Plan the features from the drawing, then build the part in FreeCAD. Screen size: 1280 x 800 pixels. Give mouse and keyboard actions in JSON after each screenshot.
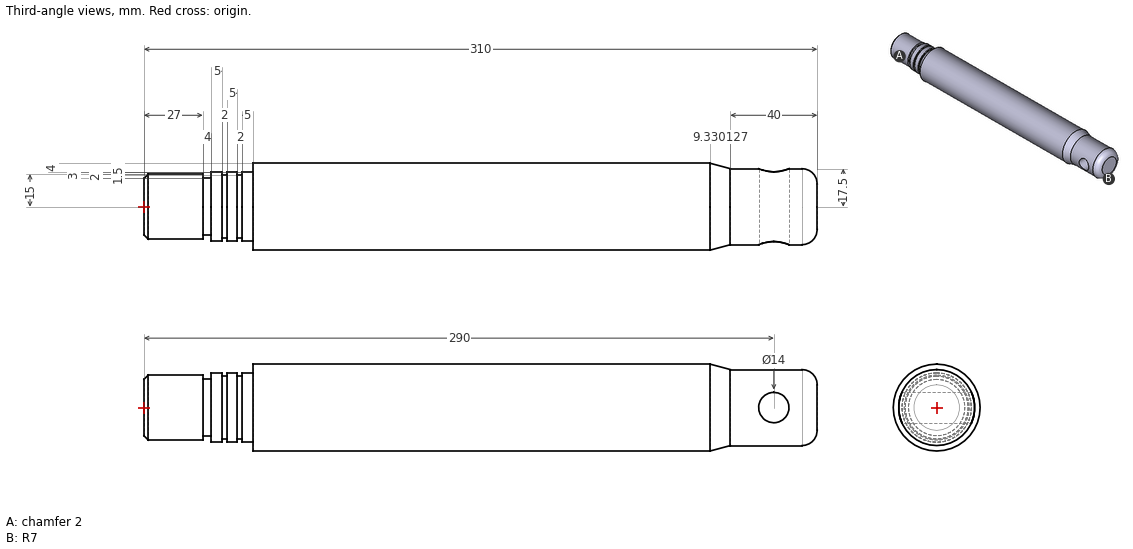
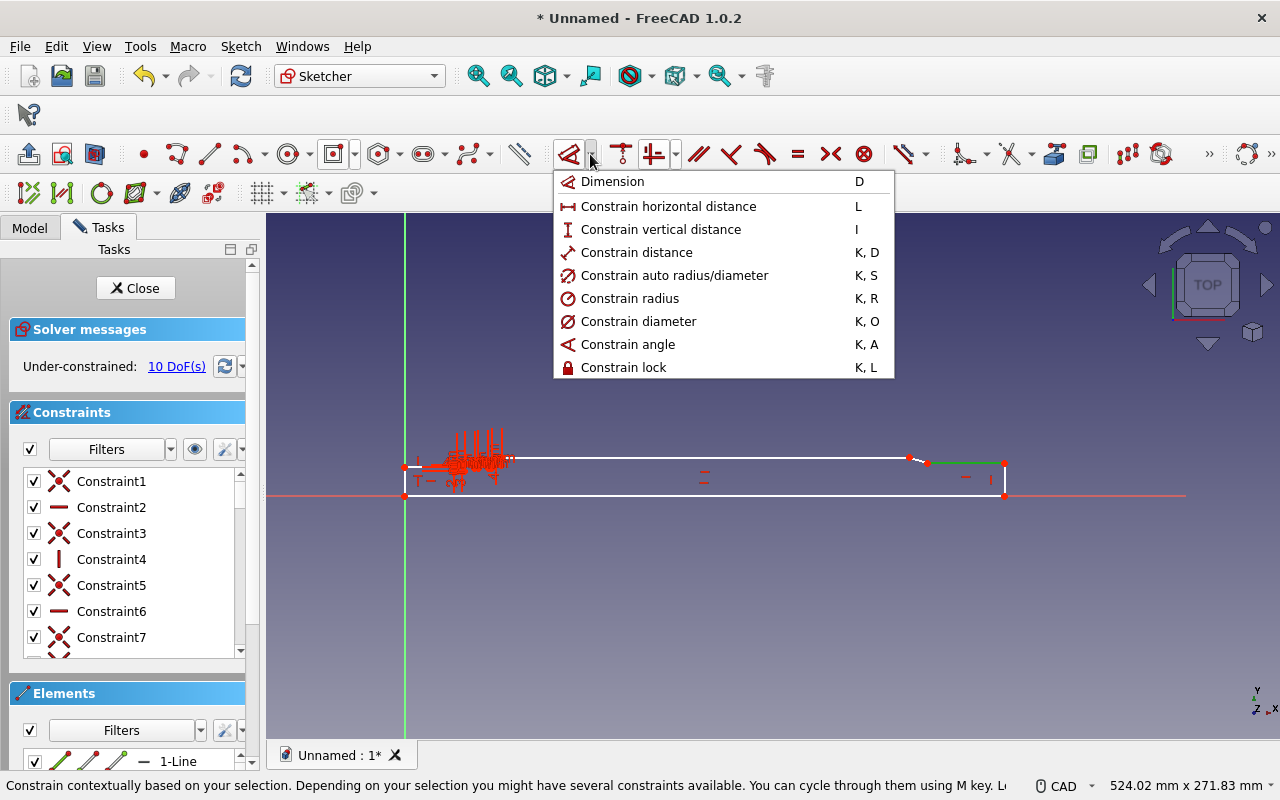
{"action": "left_click", "coordinate": [724, 206]}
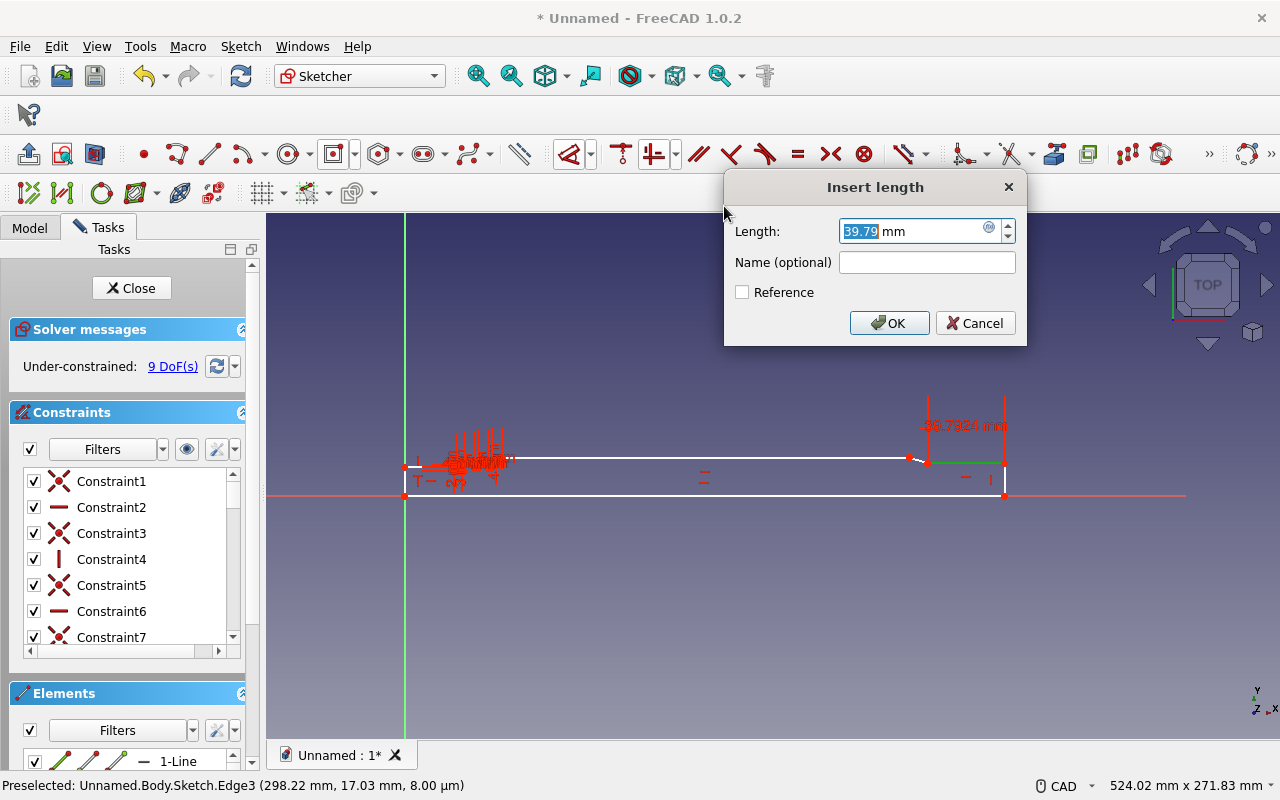
{"action": "type", "text": "40"}
{"action": "key", "text": "Return"}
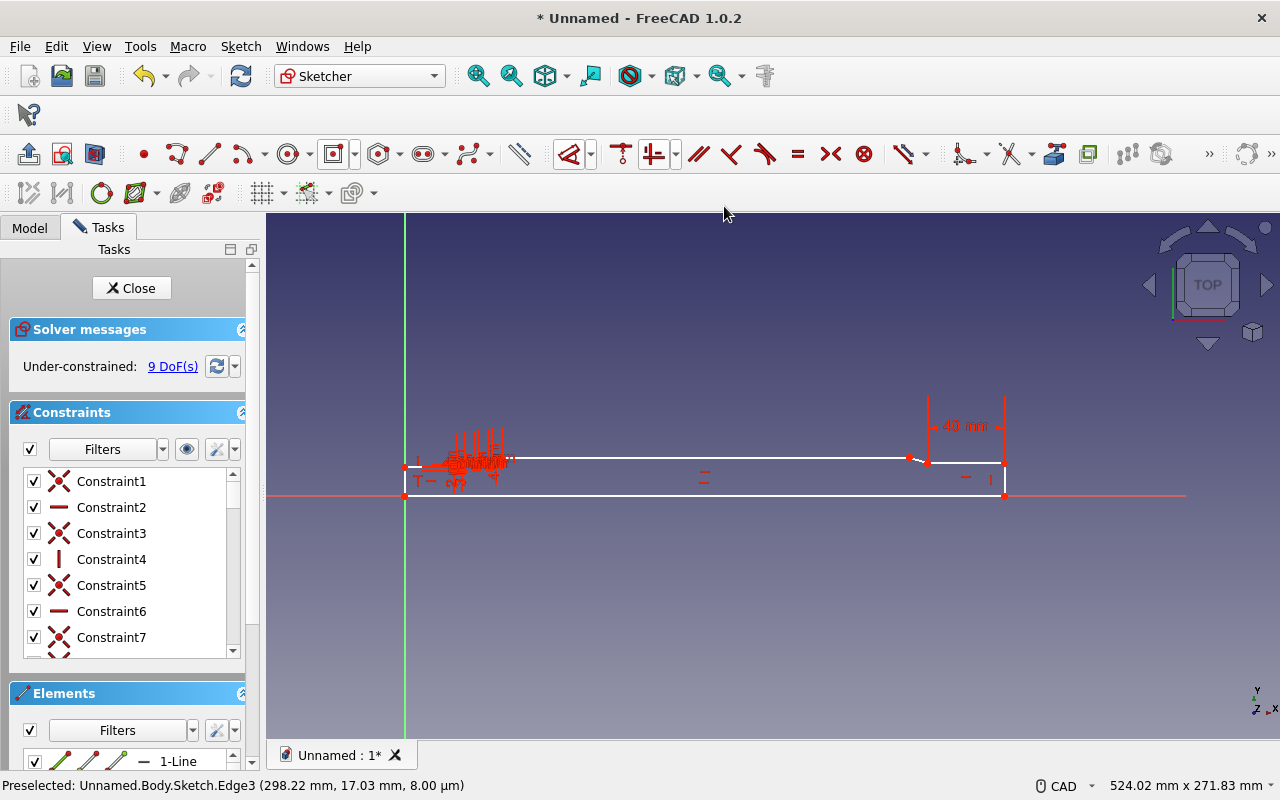
{"action": "scroll", "coordinate": [441, 467], "scroll_direction": "up", "scroll_amount": 4}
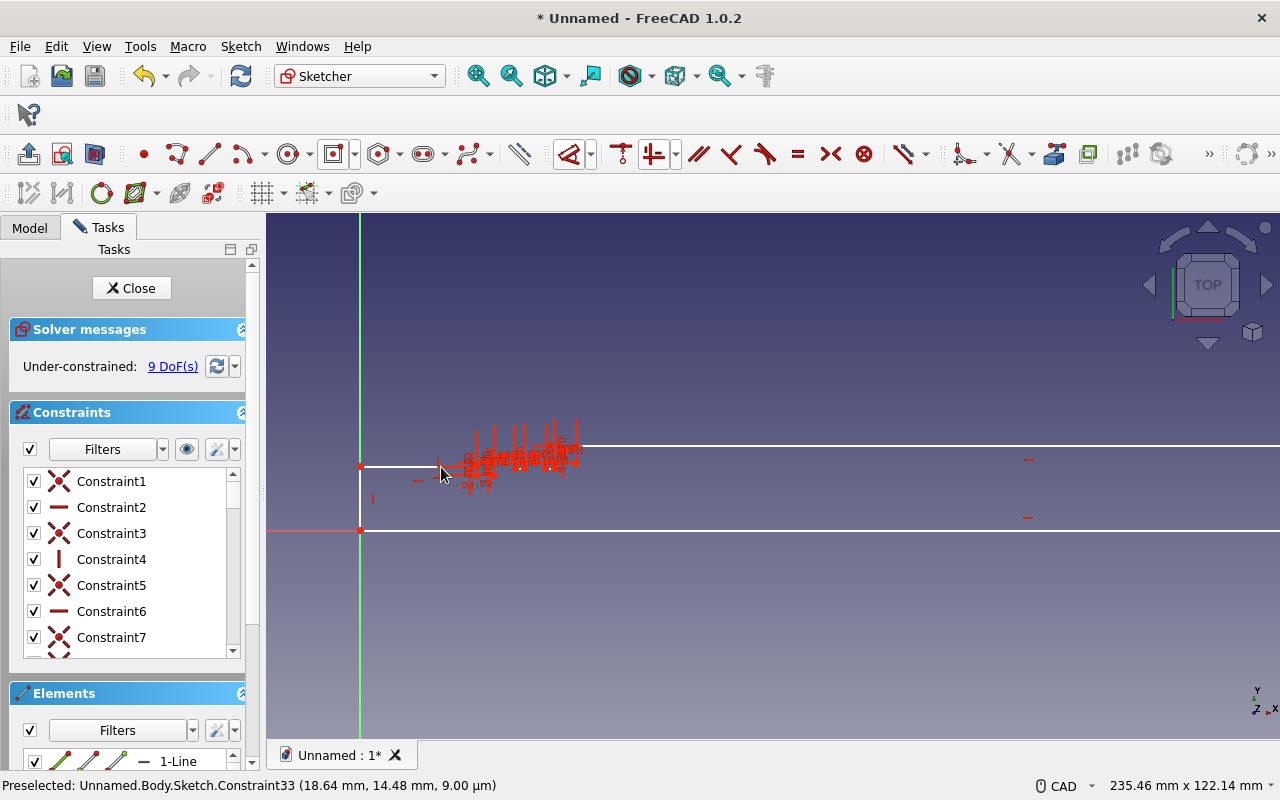
{"action": "left_click", "coordinate": [395, 467]}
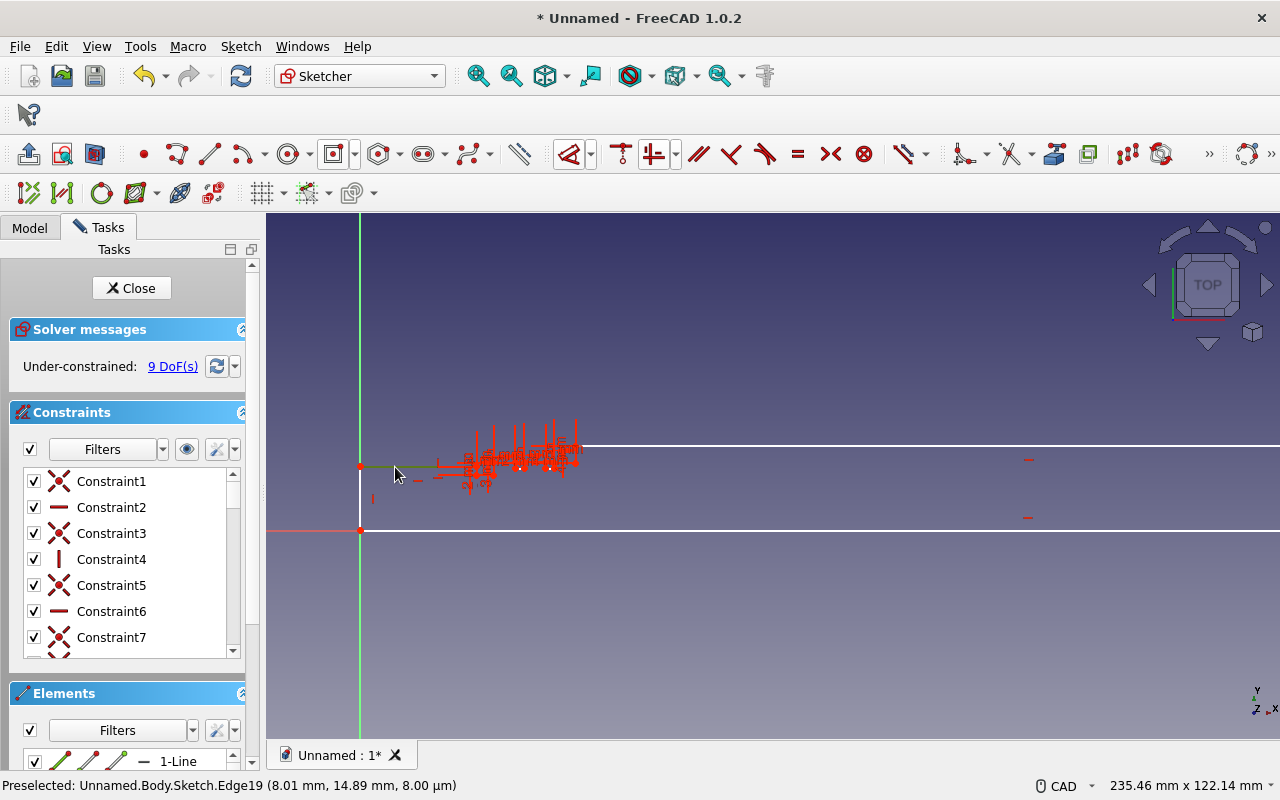
{"action": "left_click", "coordinate": [590, 154]}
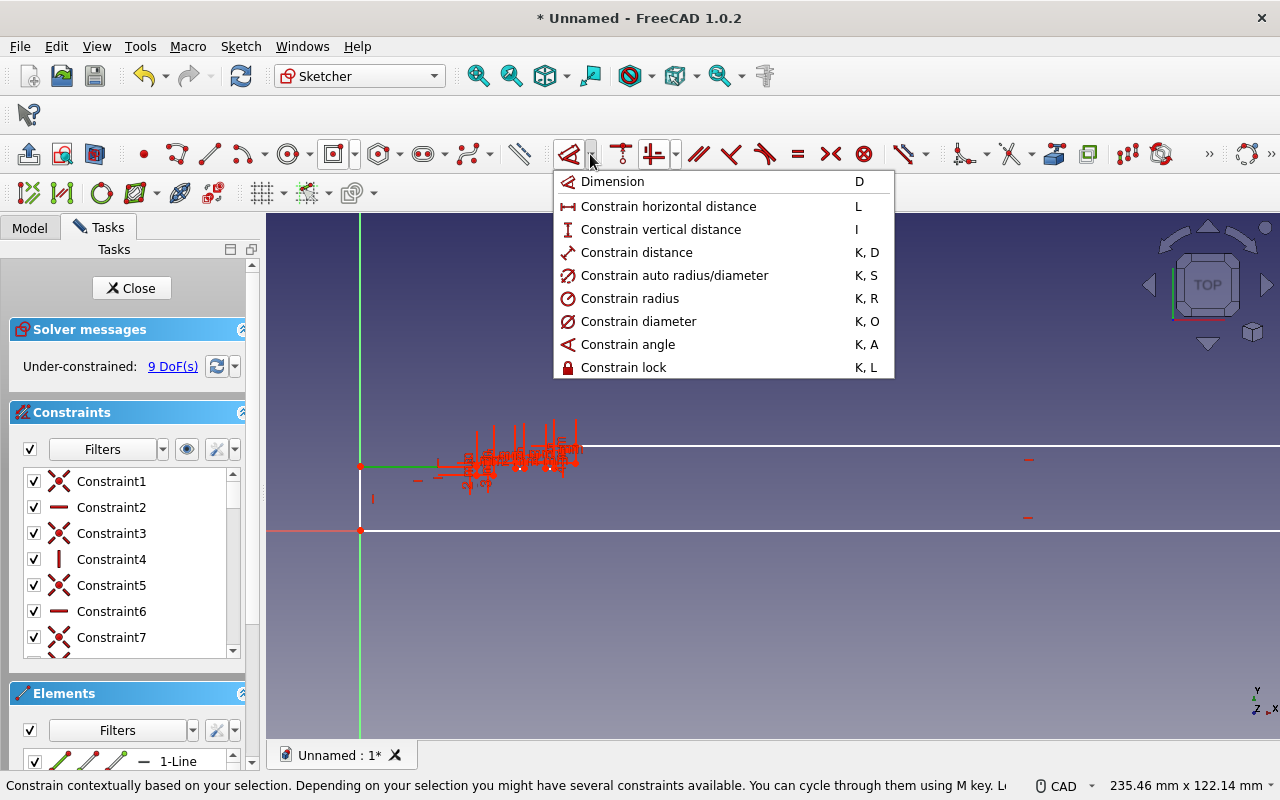
{"action": "left_click", "coordinate": [724, 206]}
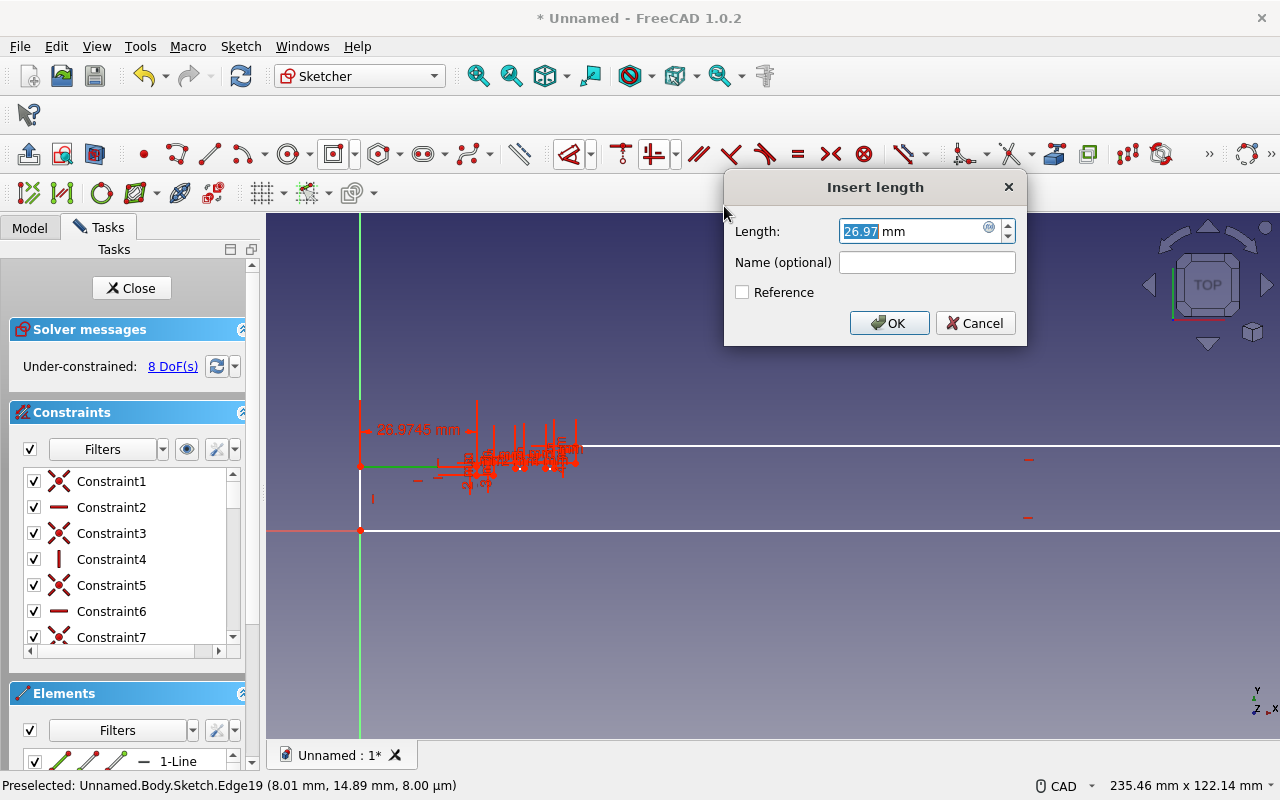
{"action": "type", "text": "27"}
{"action": "key", "text": "Return"}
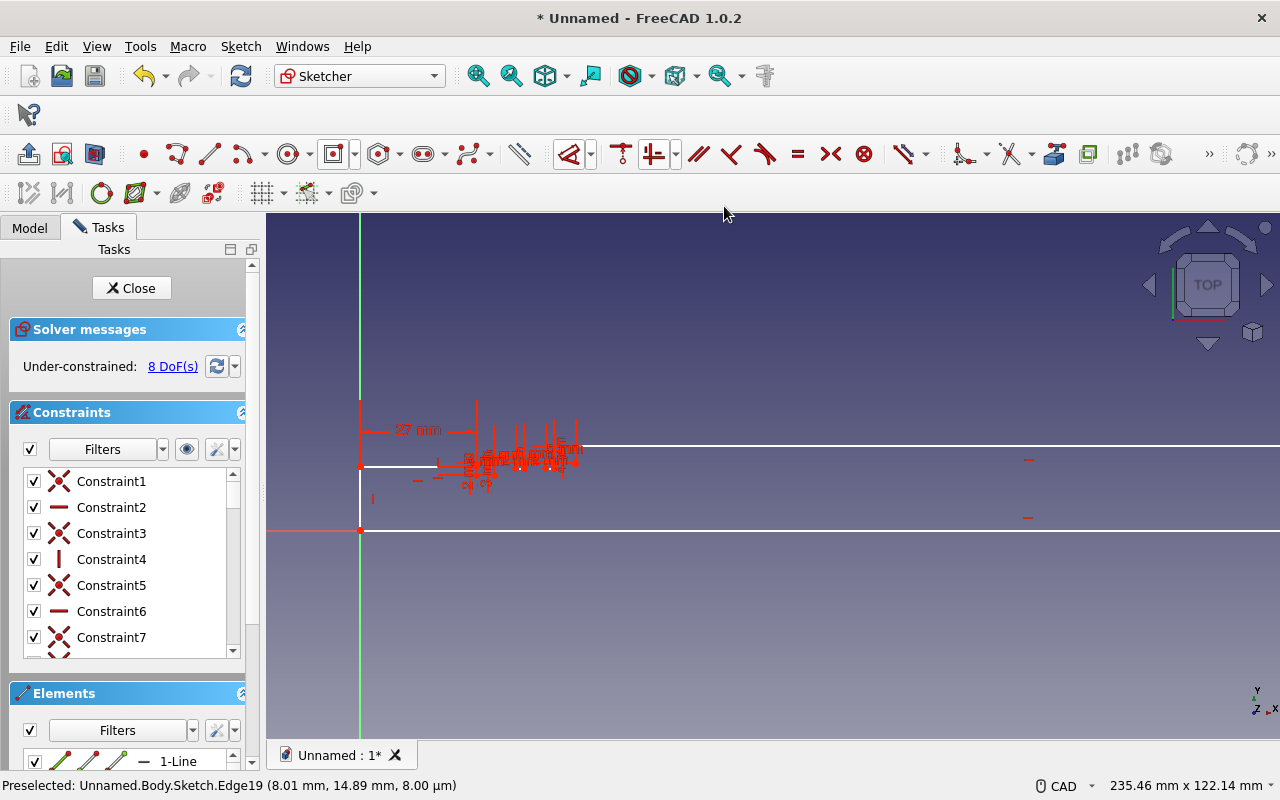
{"action": "left_click", "coordinate": [361, 486]}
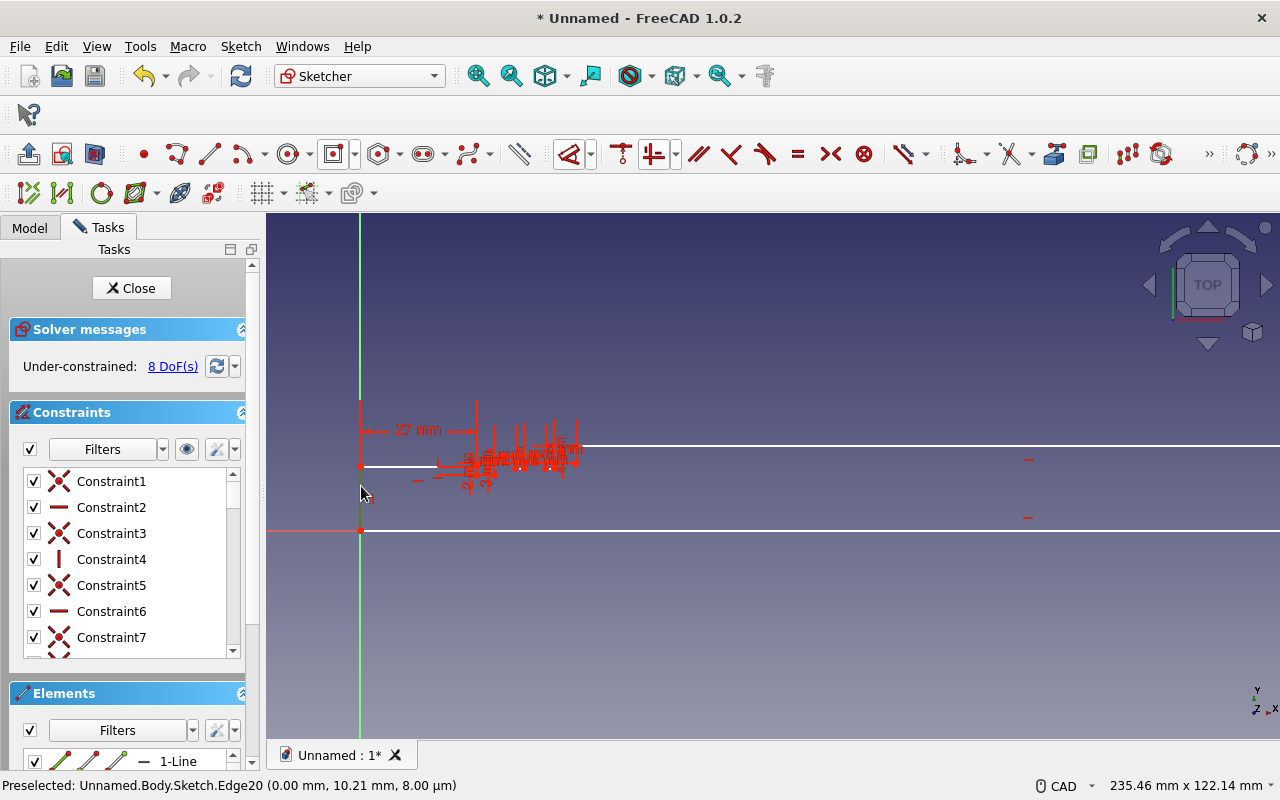
{"action": "key", "text": "i"}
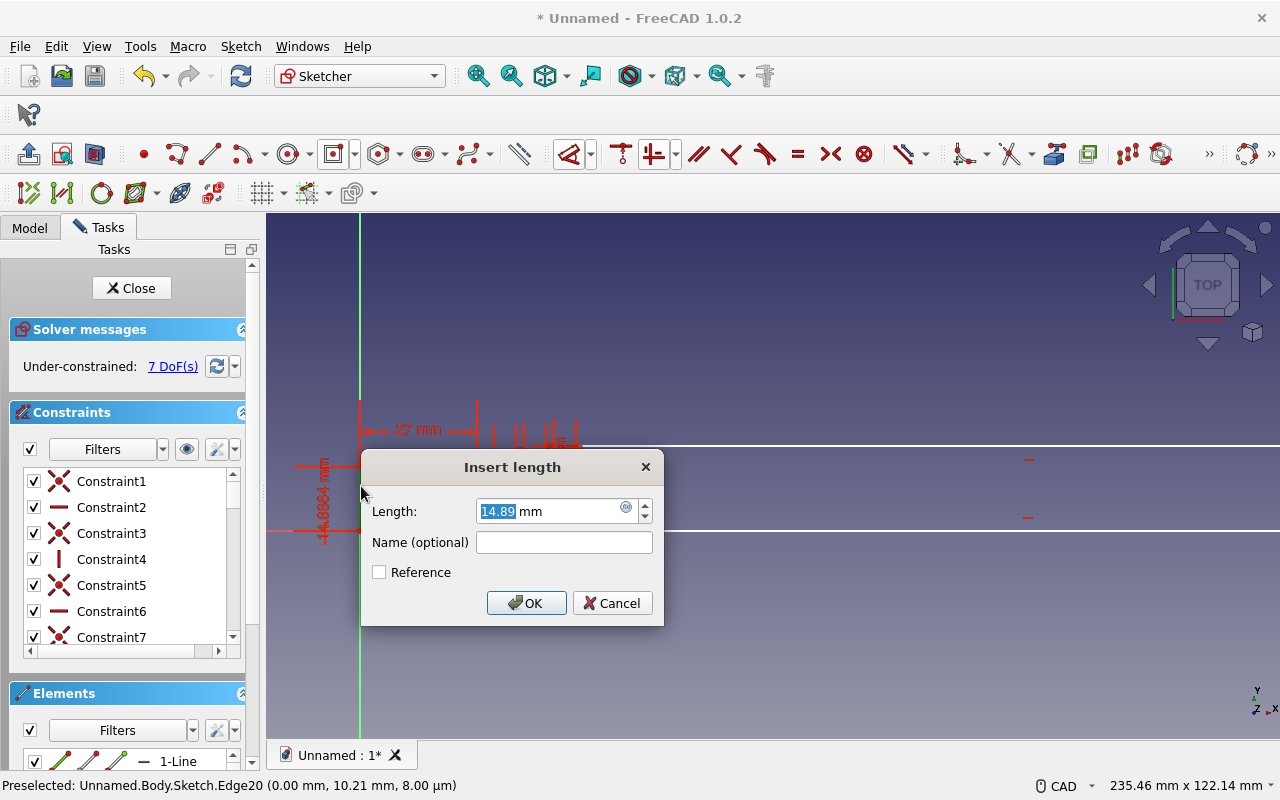
{"action": "type", "text": "15"}
{"action": "key", "text": "Return"}